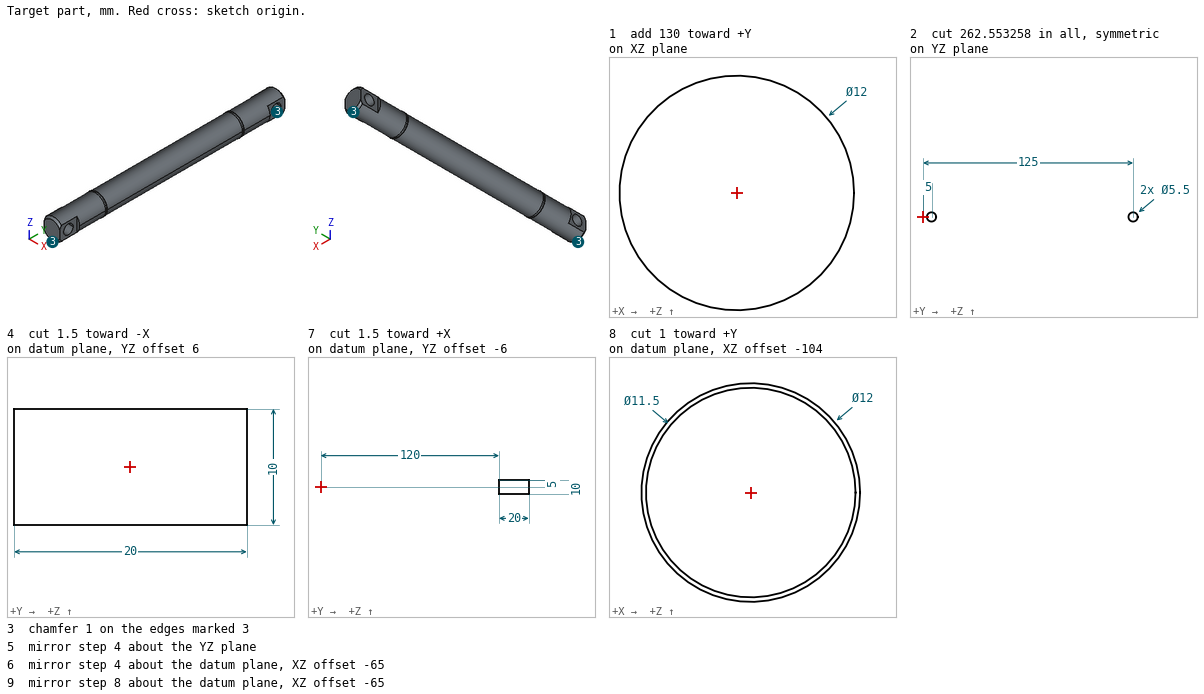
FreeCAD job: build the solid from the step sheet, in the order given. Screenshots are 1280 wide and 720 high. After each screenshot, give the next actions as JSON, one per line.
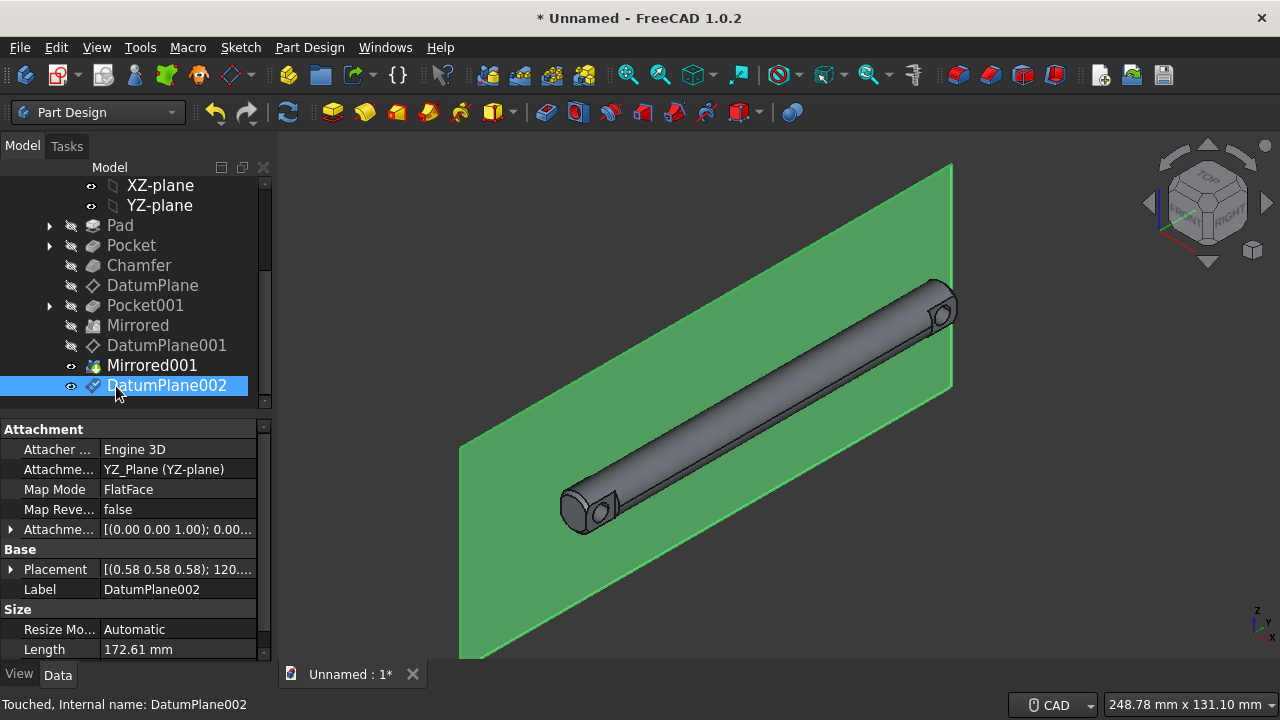
{"action": "left_click", "coordinate": [58, 76]}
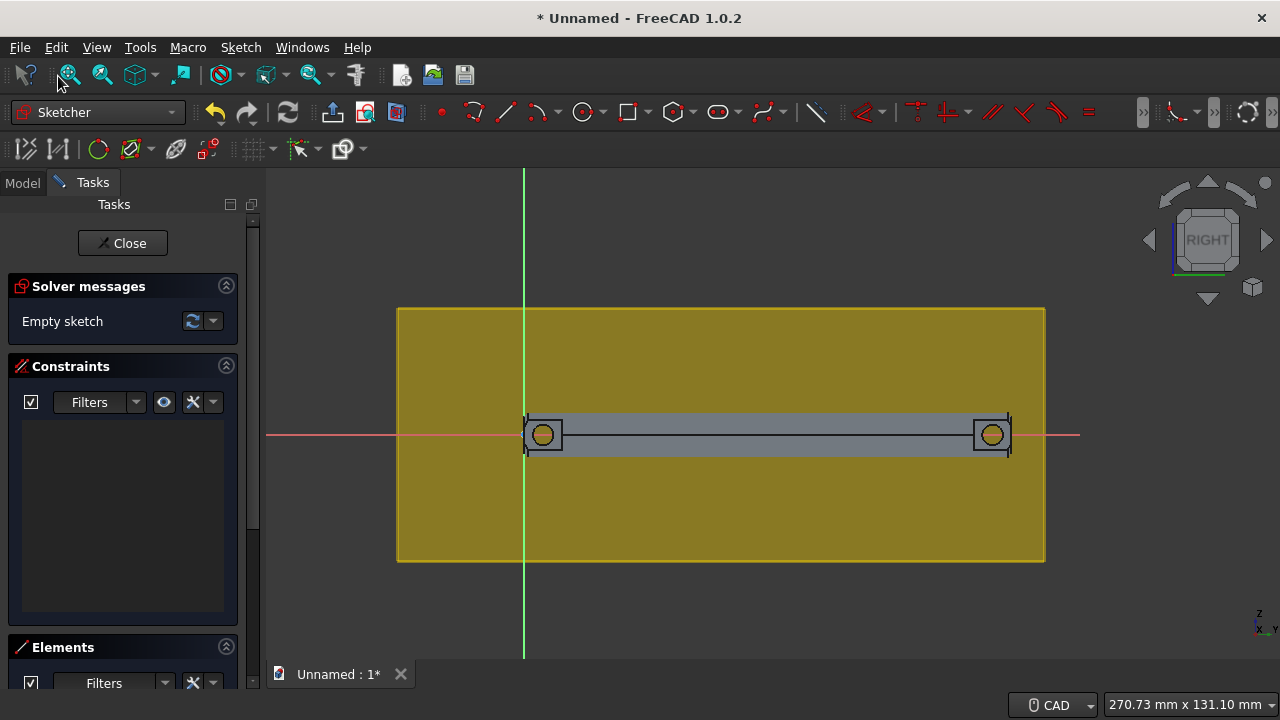
{"action": "key", "text": "q s"}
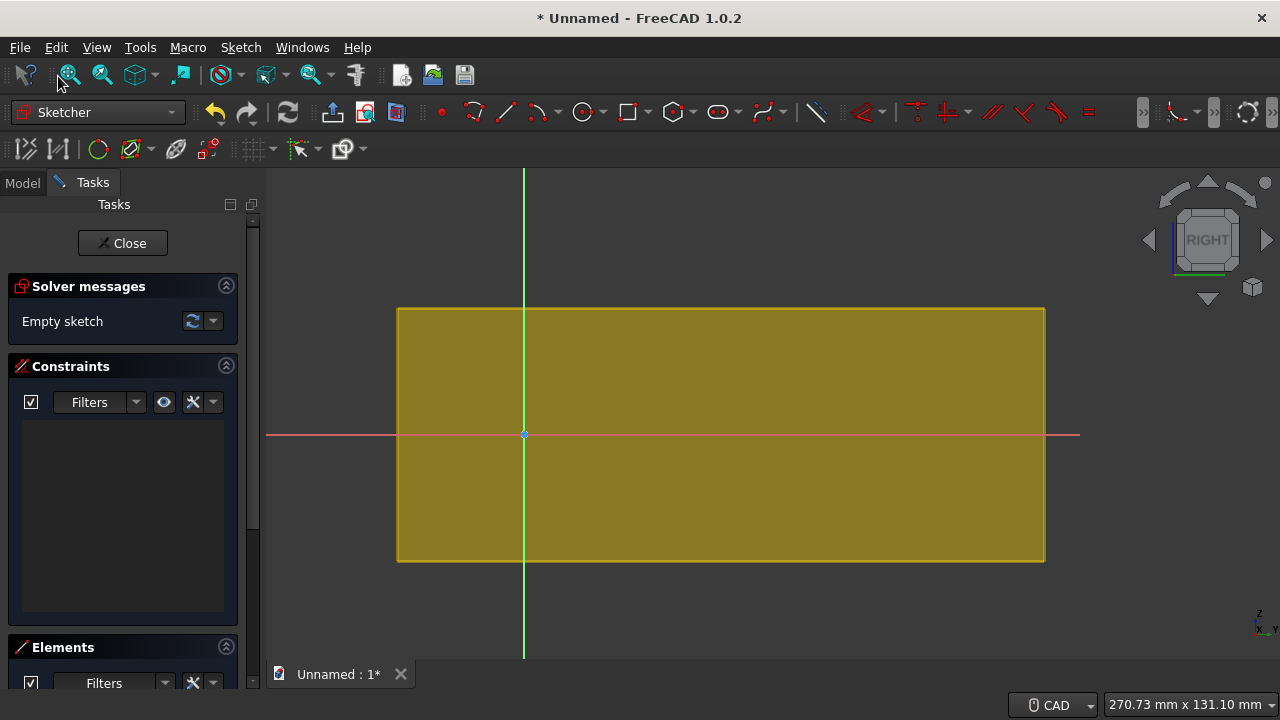
{"action": "scroll", "coordinate": [1059, 438], "scroll_direction": "up", "scroll_amount": 10}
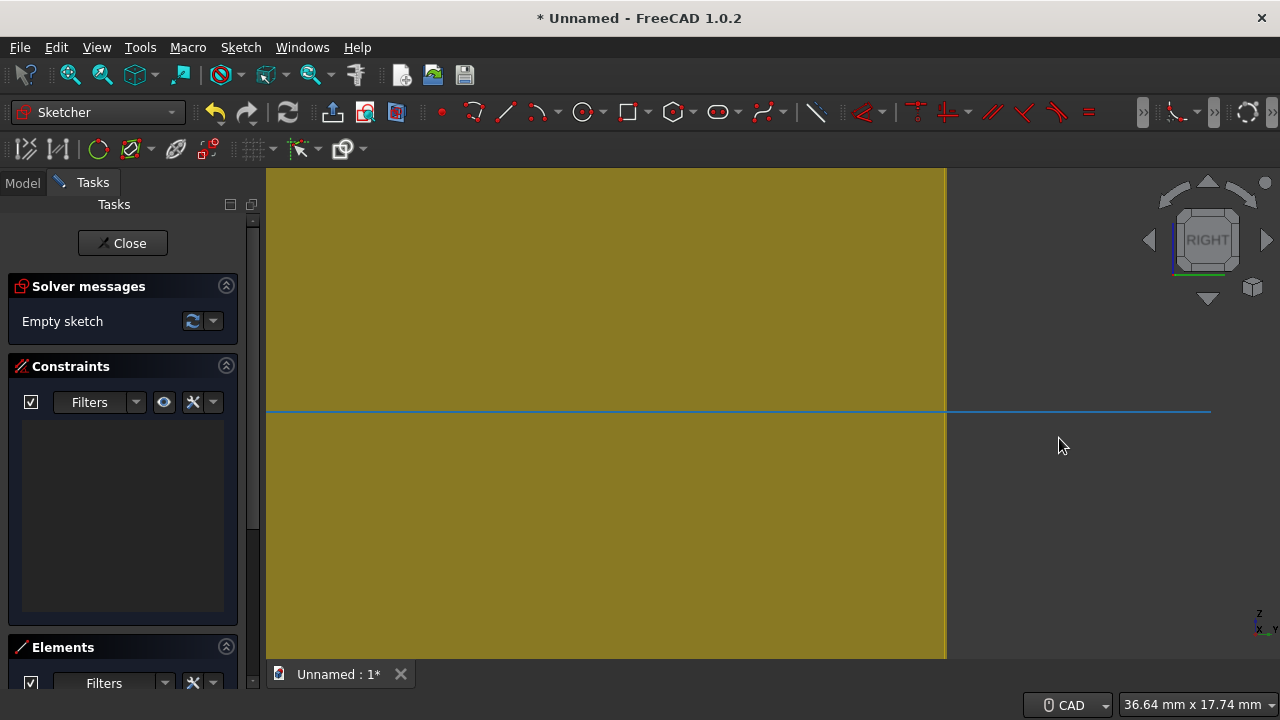
{"action": "key", "text": "g r"}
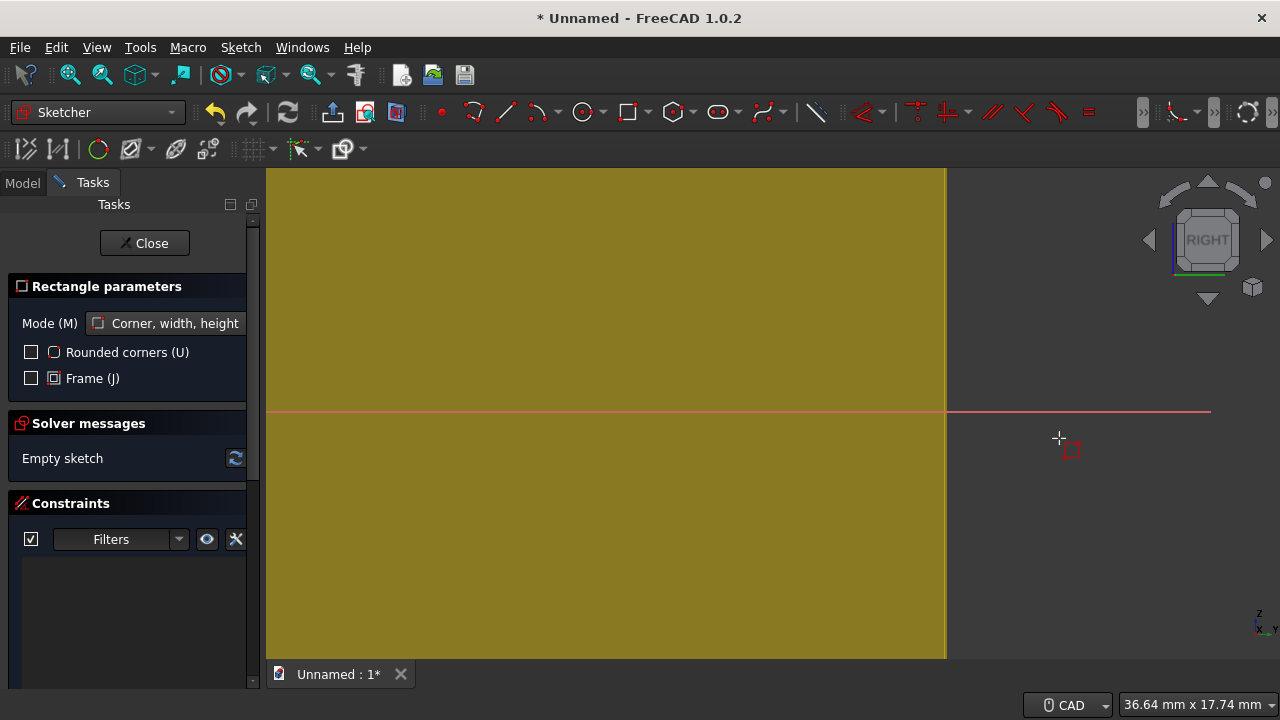
{"action": "left_click", "coordinate": [425, 274]}
{"action": "mouse_move", "coordinate": [978, 550]}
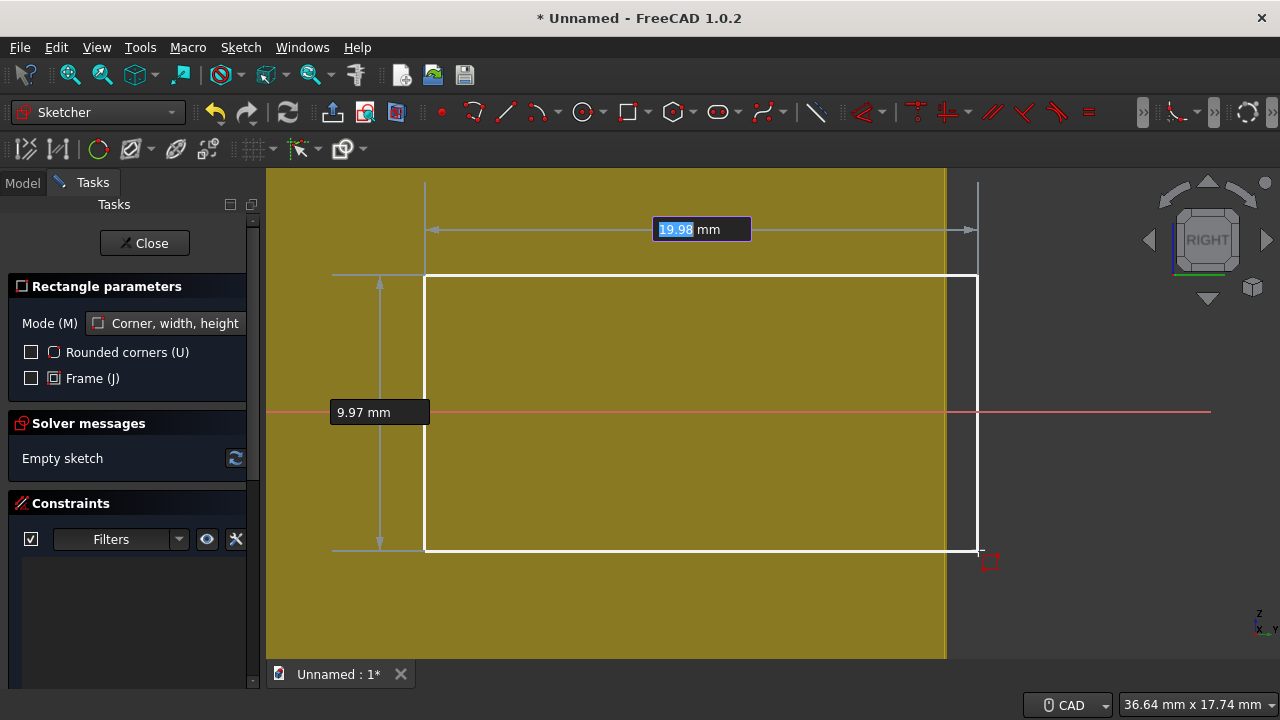
{"action": "type", "text": "20"}
{"action": "key", "text": "Tab"}
{"action": "type", "text": "10"}
{"action": "key", "text": "Return"}
{"action": "key", "text": "Escape"}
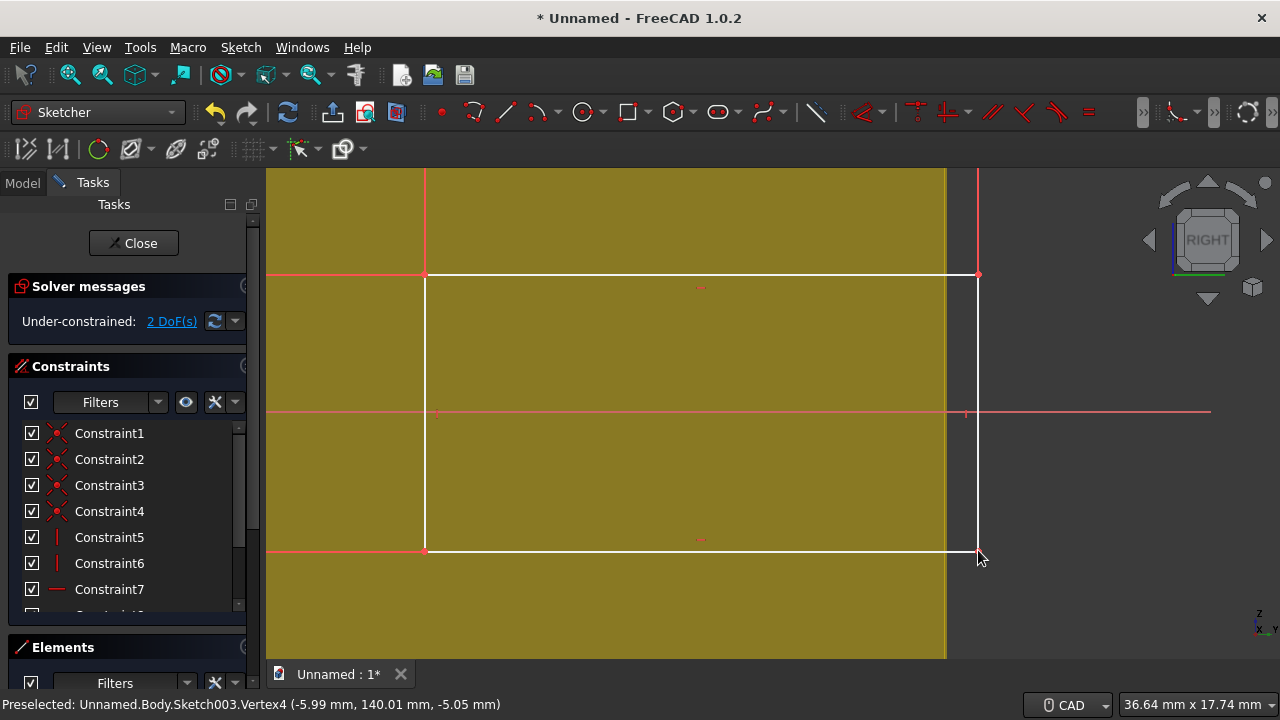
{"action": "left_click", "coordinate": [862, 112]}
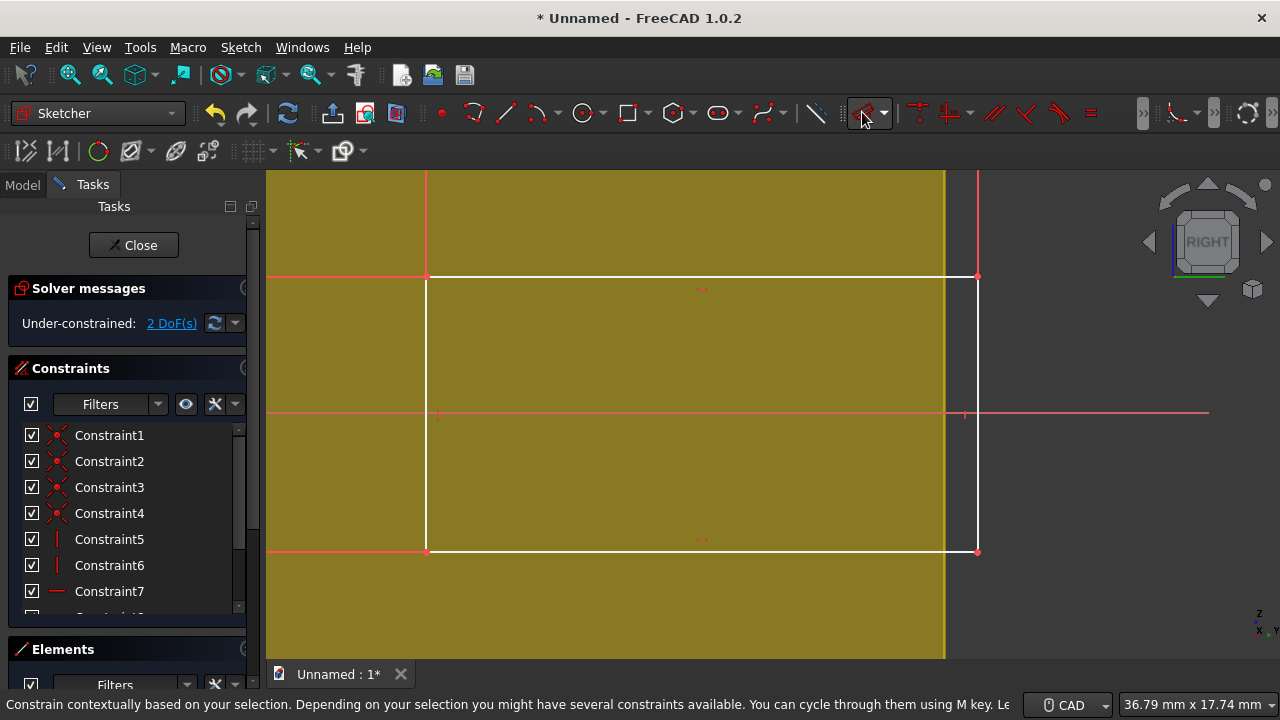
{"action": "left_click", "coordinate": [426, 277]}
{"action": "left_click", "coordinate": [460, 345]}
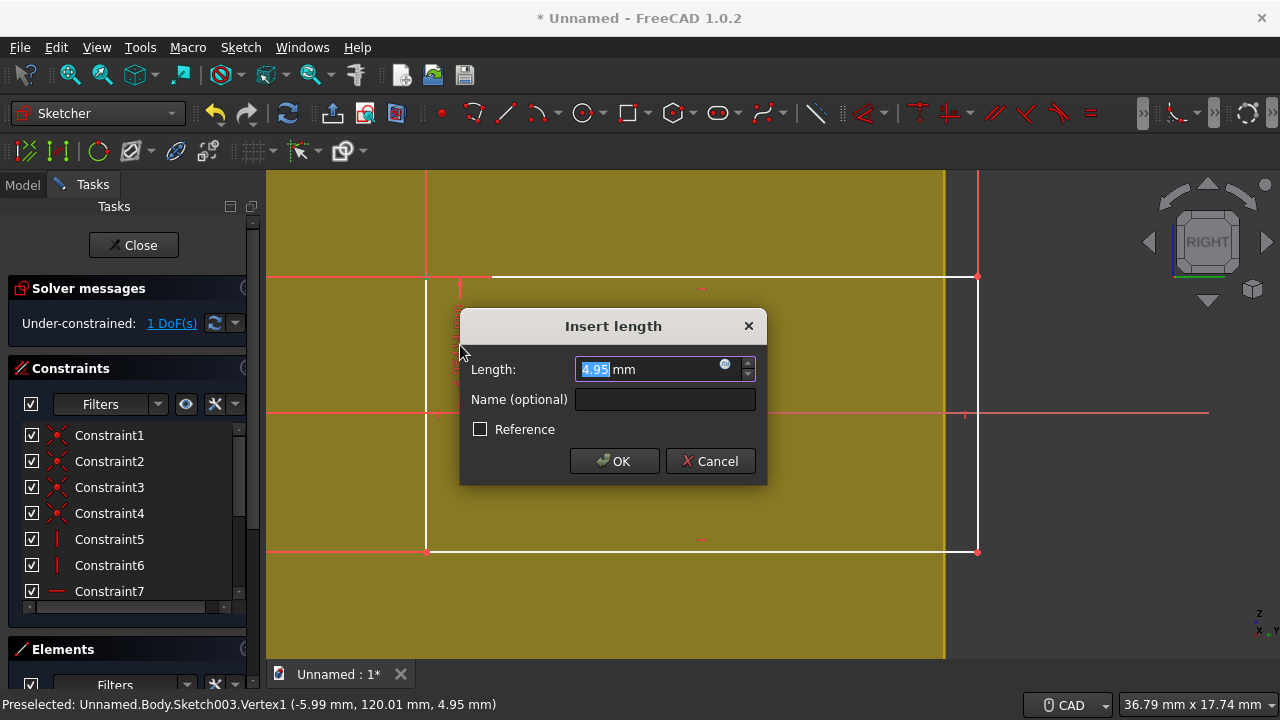
{"action": "type", "text": "5"}
{"action": "key", "text": "Return"}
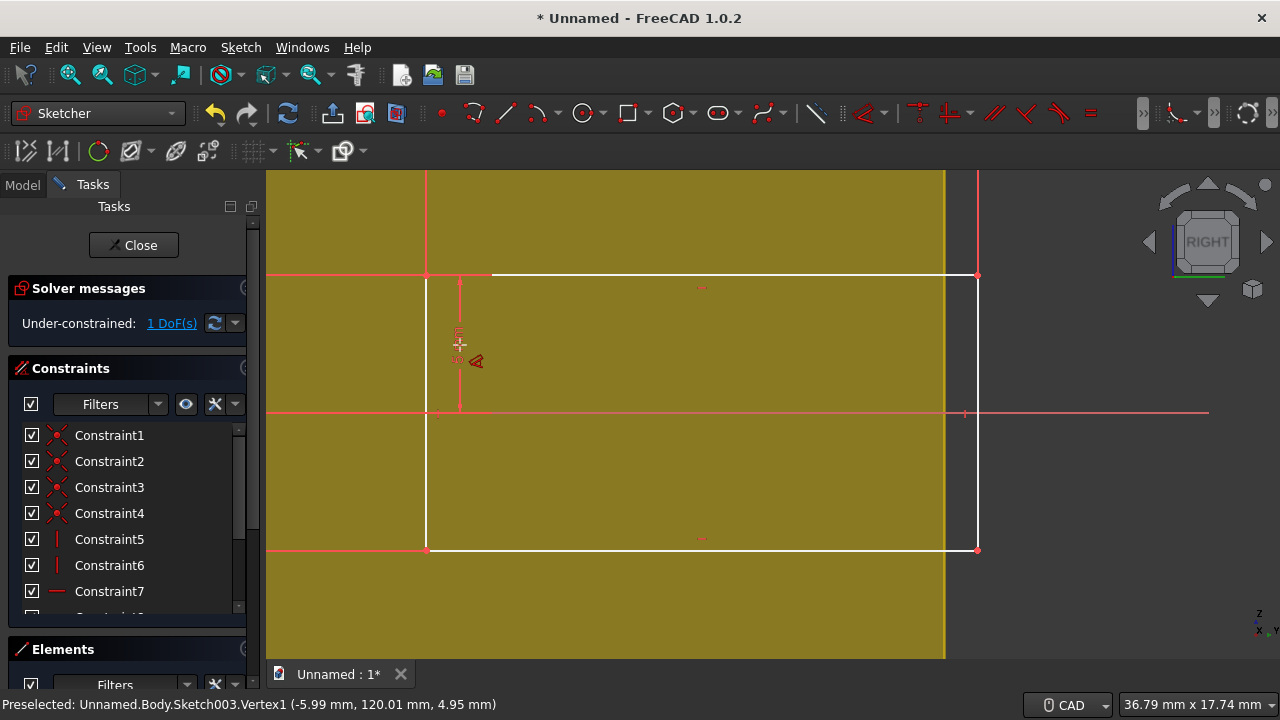
{"action": "left_click", "coordinate": [426, 275]}
{"action": "left_click", "coordinate": [360, 241]}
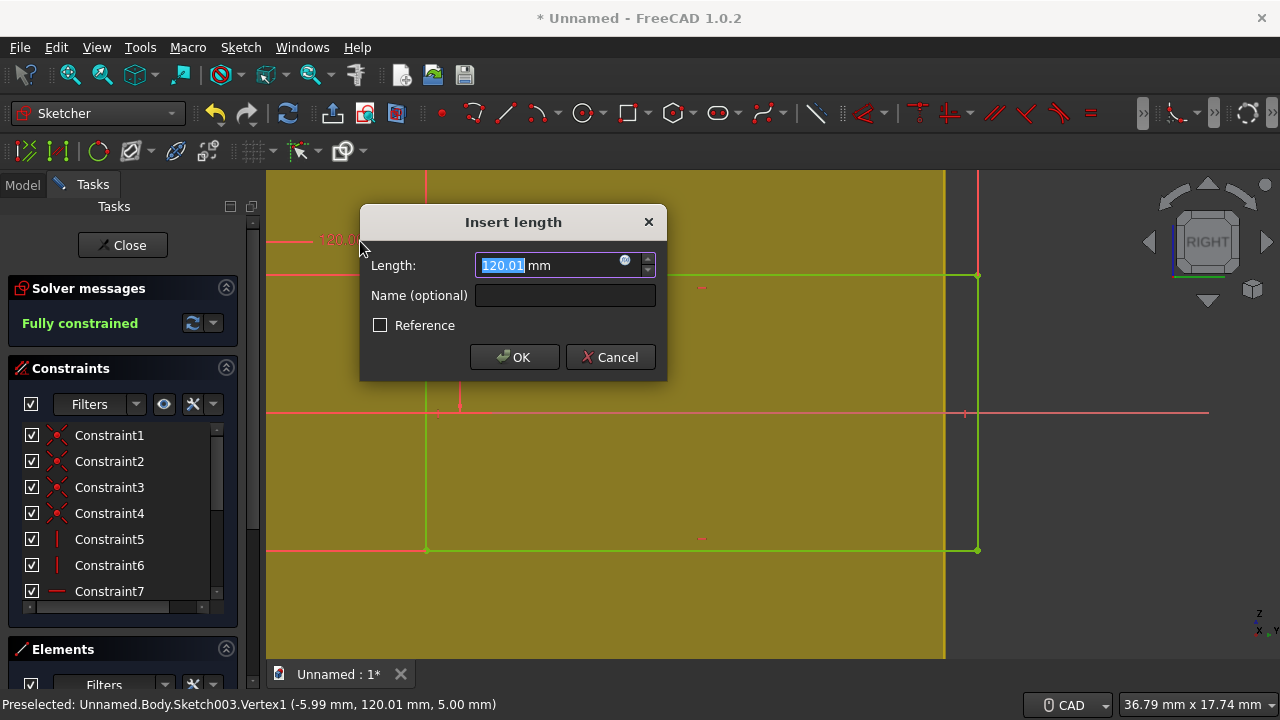
{"action": "type", "text": "120"}
{"action": "key", "text": "Return"}
{"action": "key", "text": "Escape"}